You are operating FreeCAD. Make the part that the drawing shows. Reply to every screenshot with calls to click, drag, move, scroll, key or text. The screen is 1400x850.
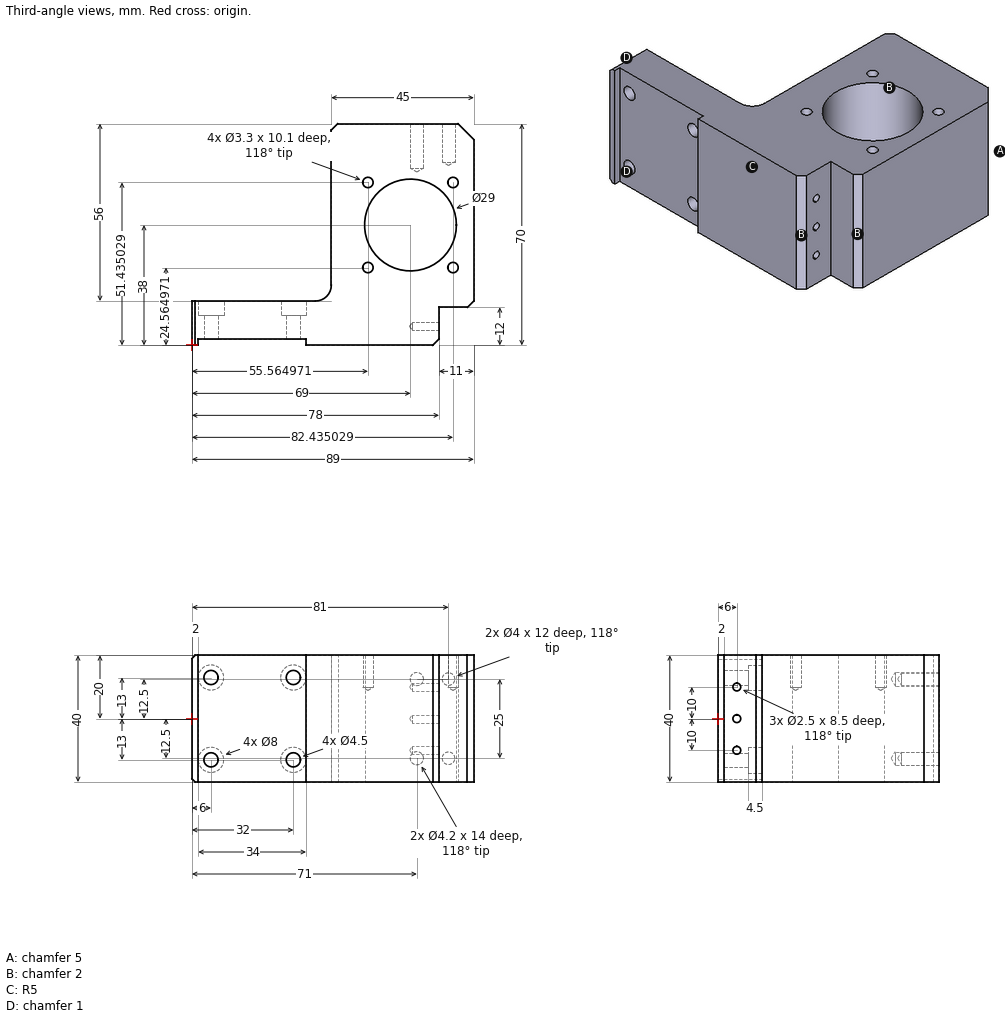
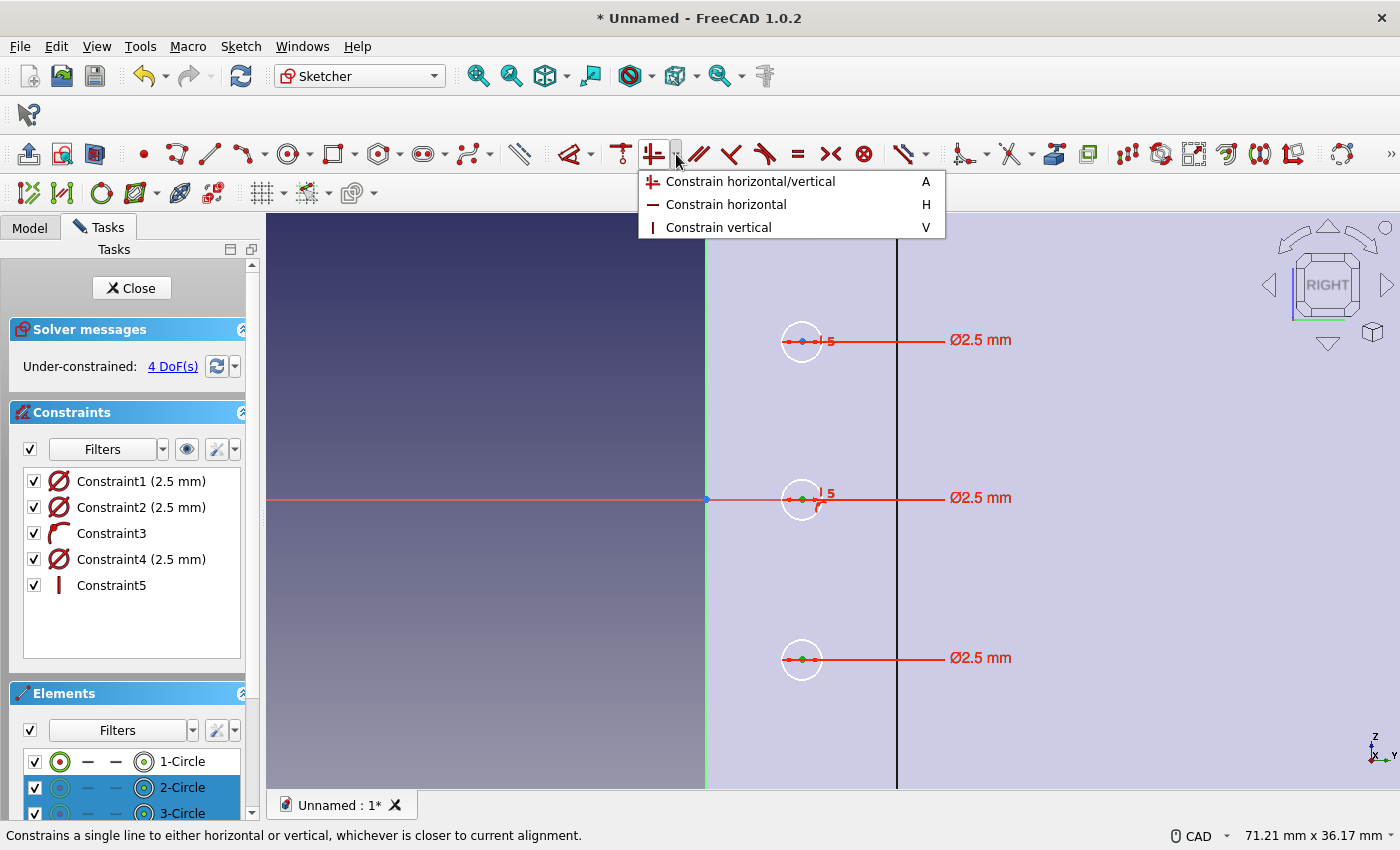
click(792, 228)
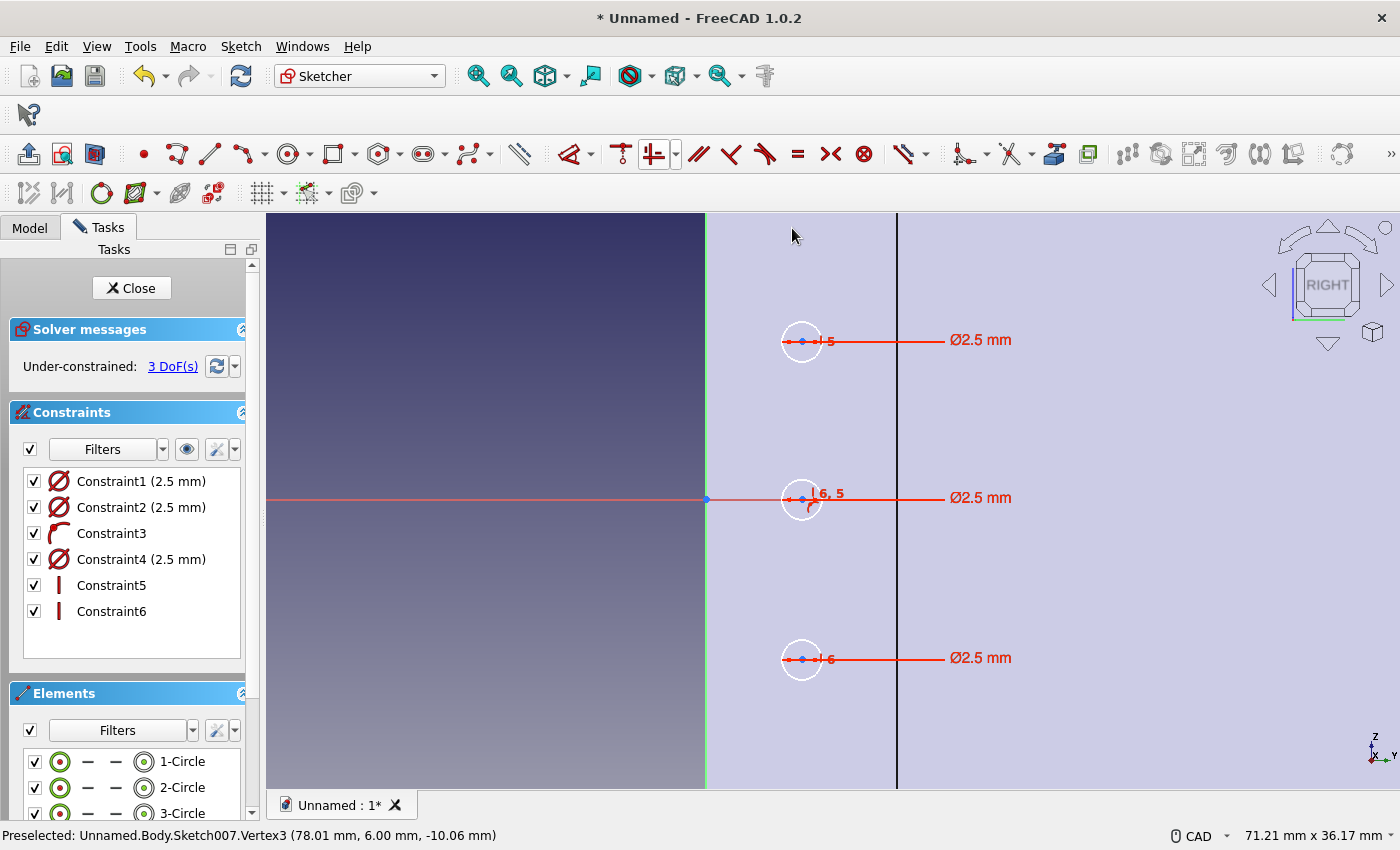
click(568, 154)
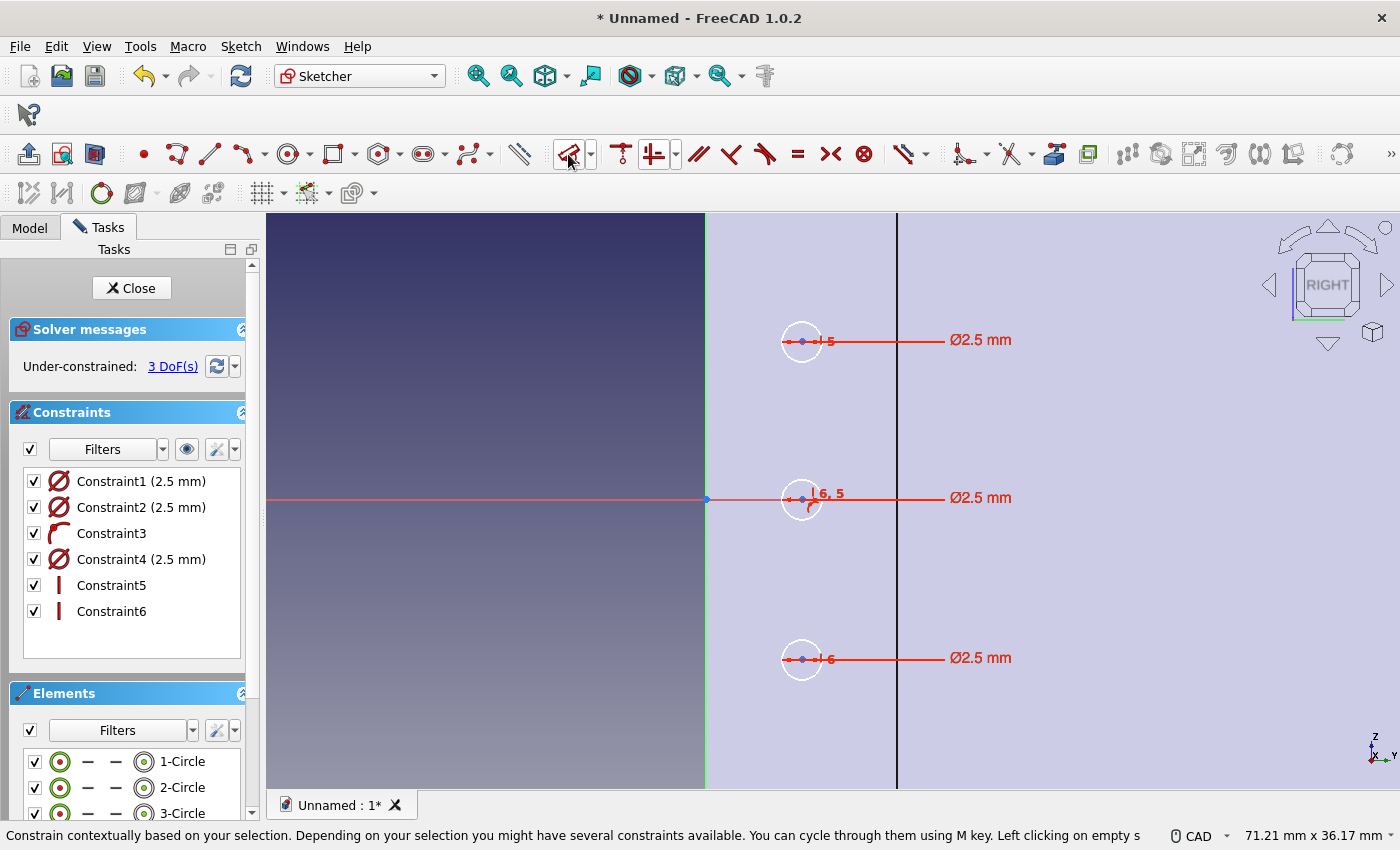
click(802, 342)
click(754, 308)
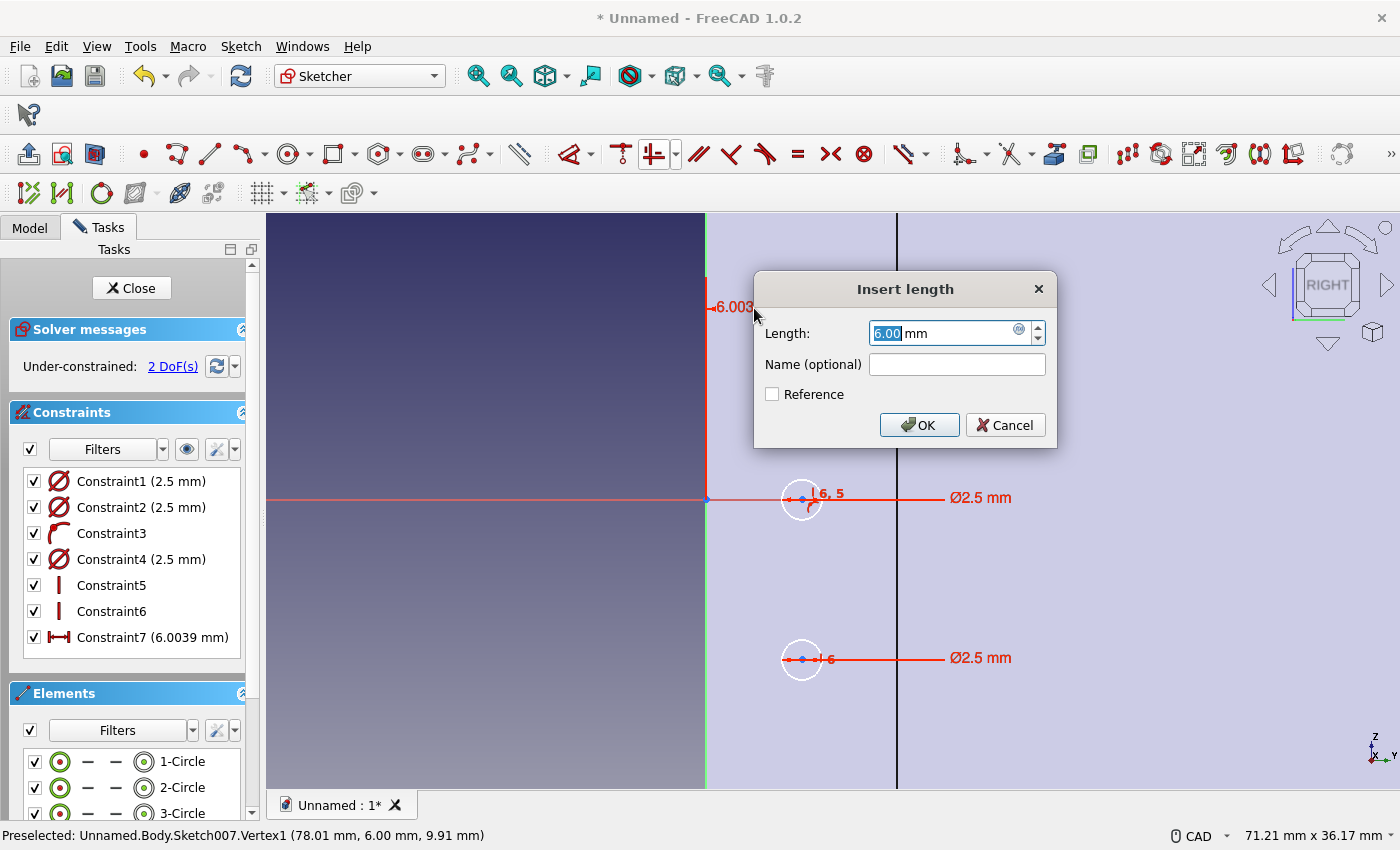
text(6)
key(Return)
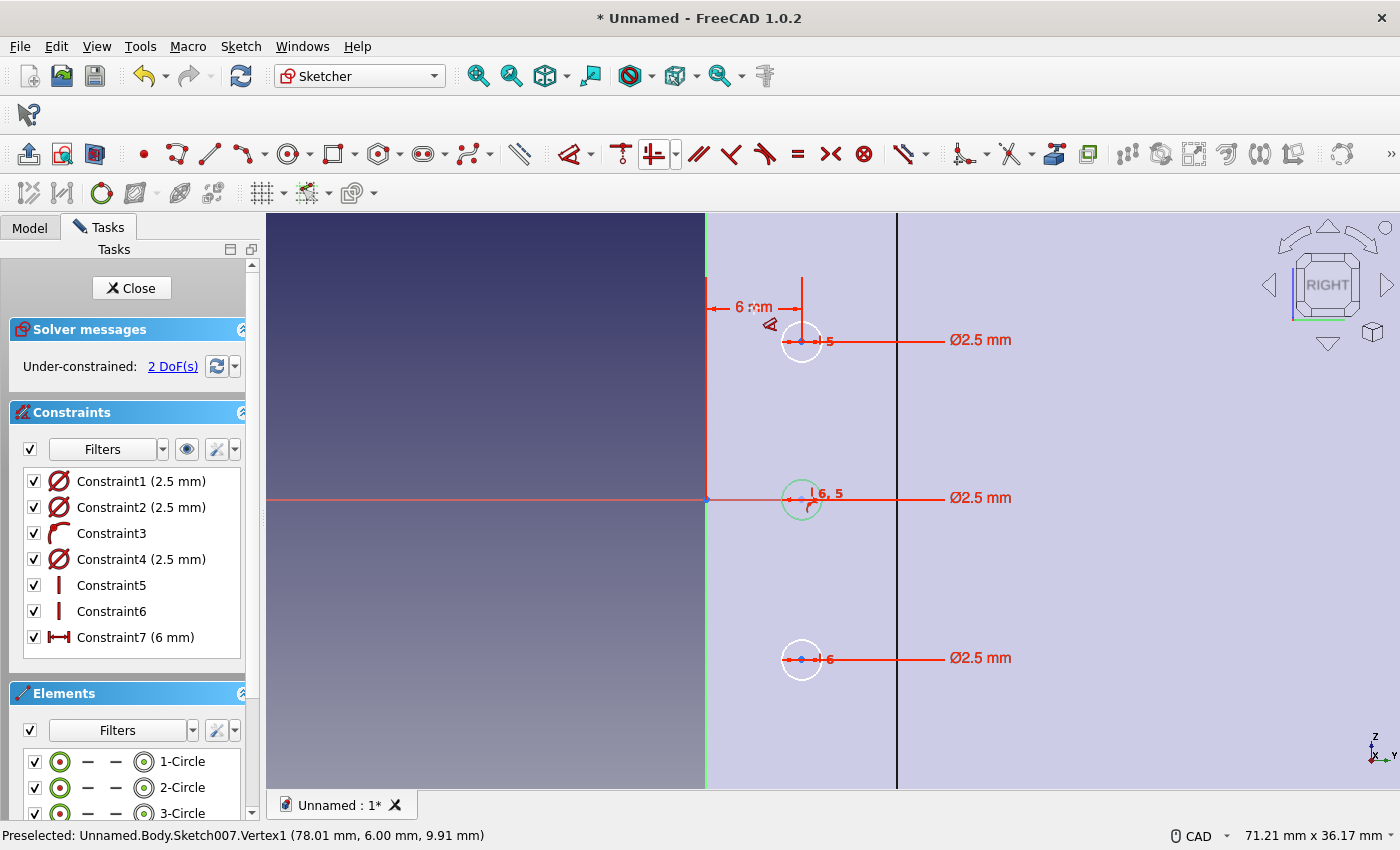
click(802, 342)
click(672, 421)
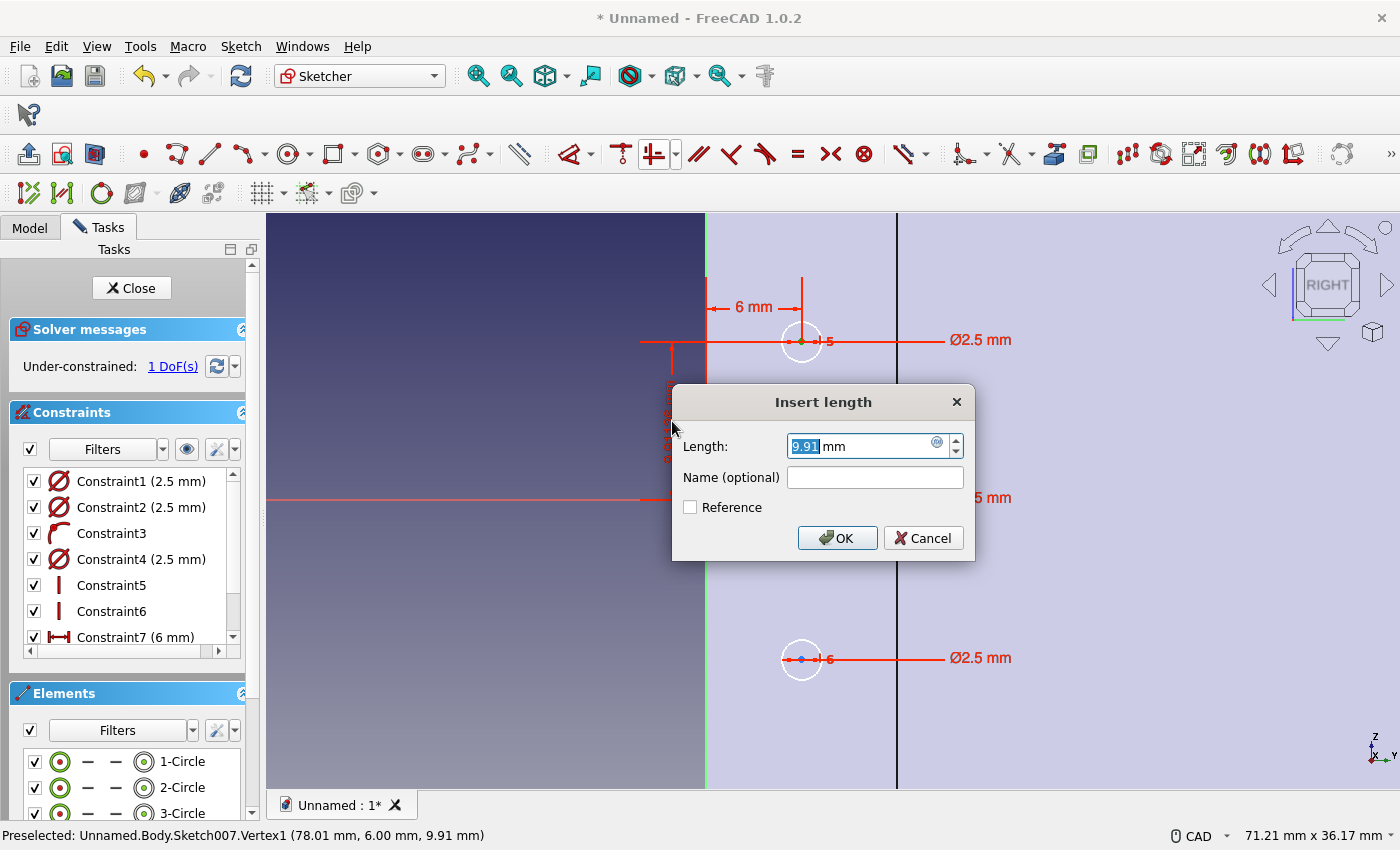
text(10)
key(Return)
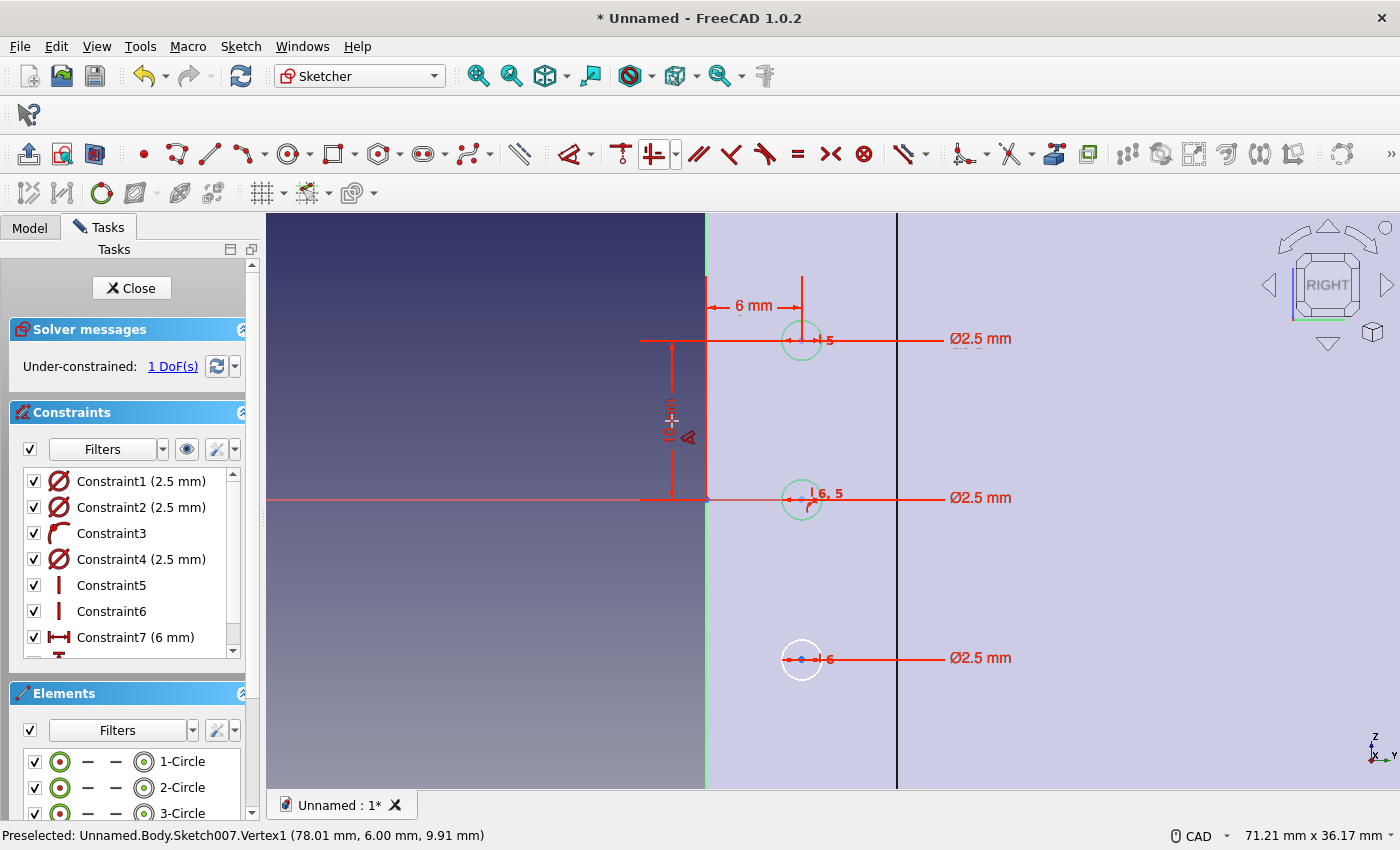
click(802, 660)
click(672, 580)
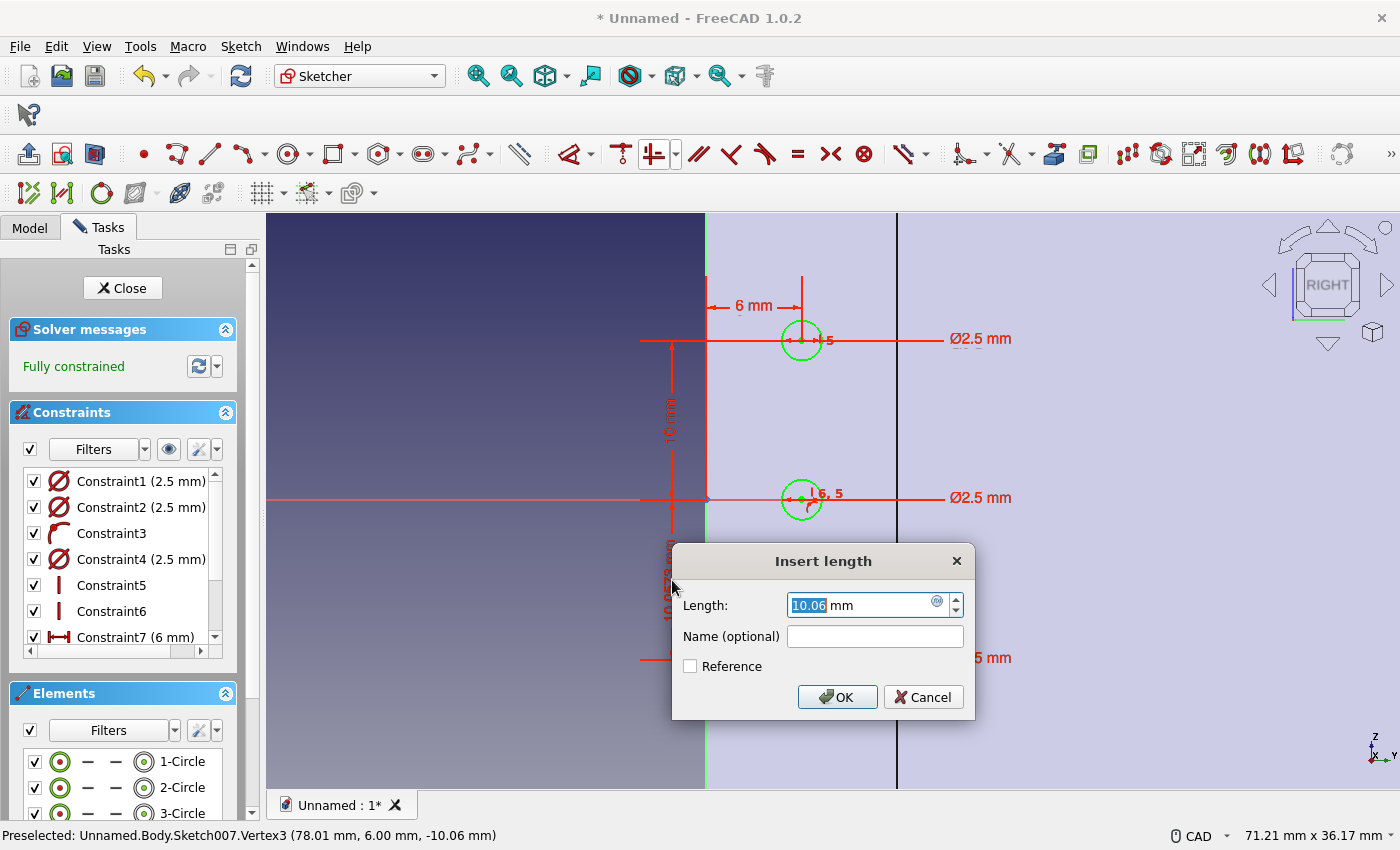
text(10)
key(Return)
key(Escape)